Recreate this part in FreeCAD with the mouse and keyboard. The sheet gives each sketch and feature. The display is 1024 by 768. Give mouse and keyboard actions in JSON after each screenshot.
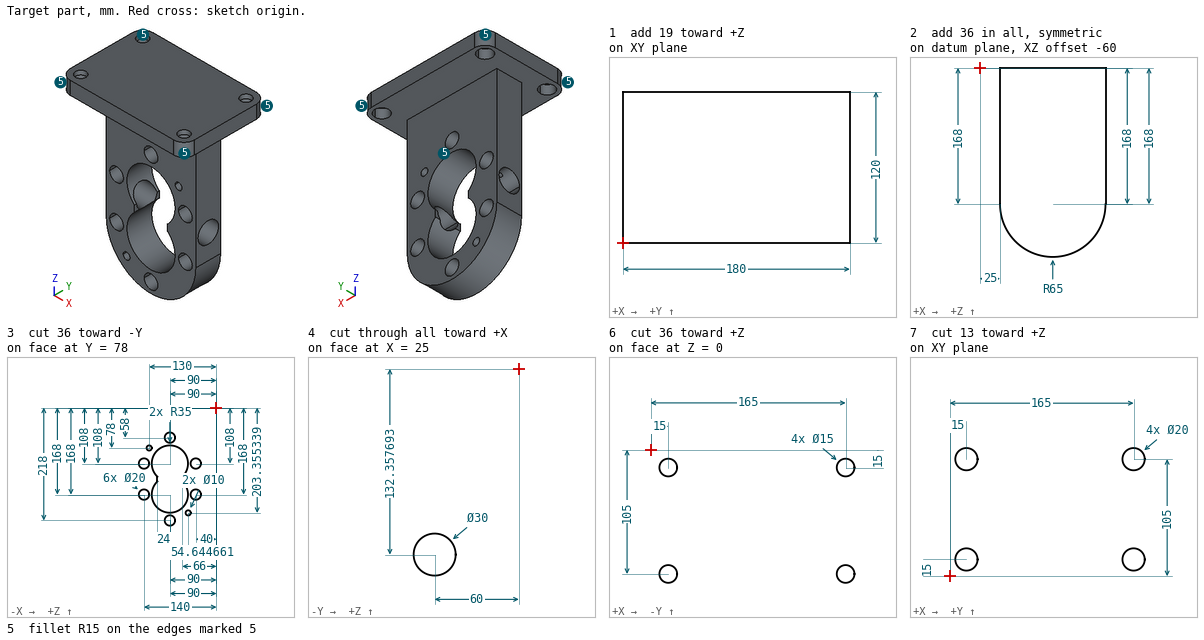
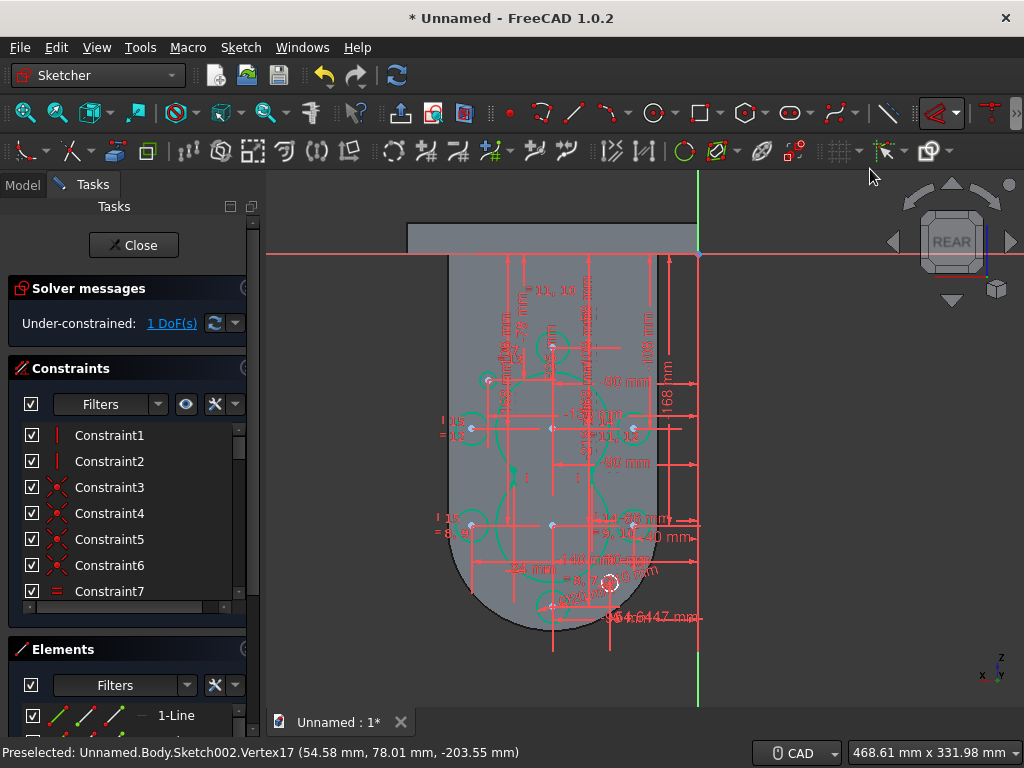
{"action": "left_click", "coordinate": [610, 583]}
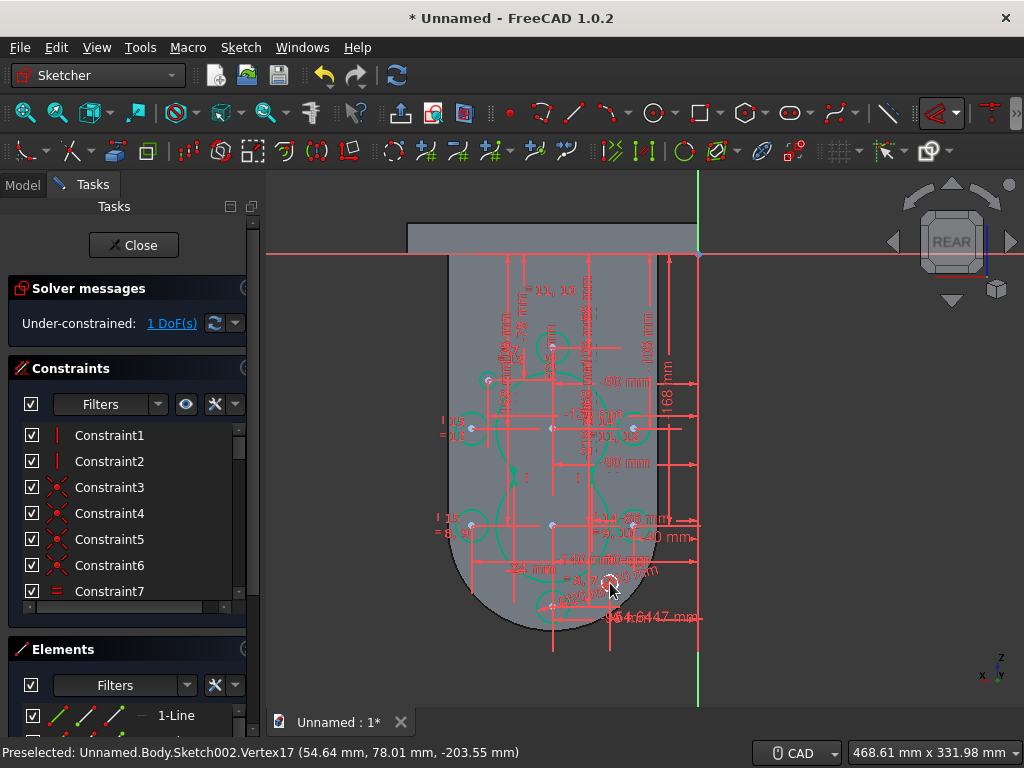
{"action": "left_click", "coordinate": [958, 114]}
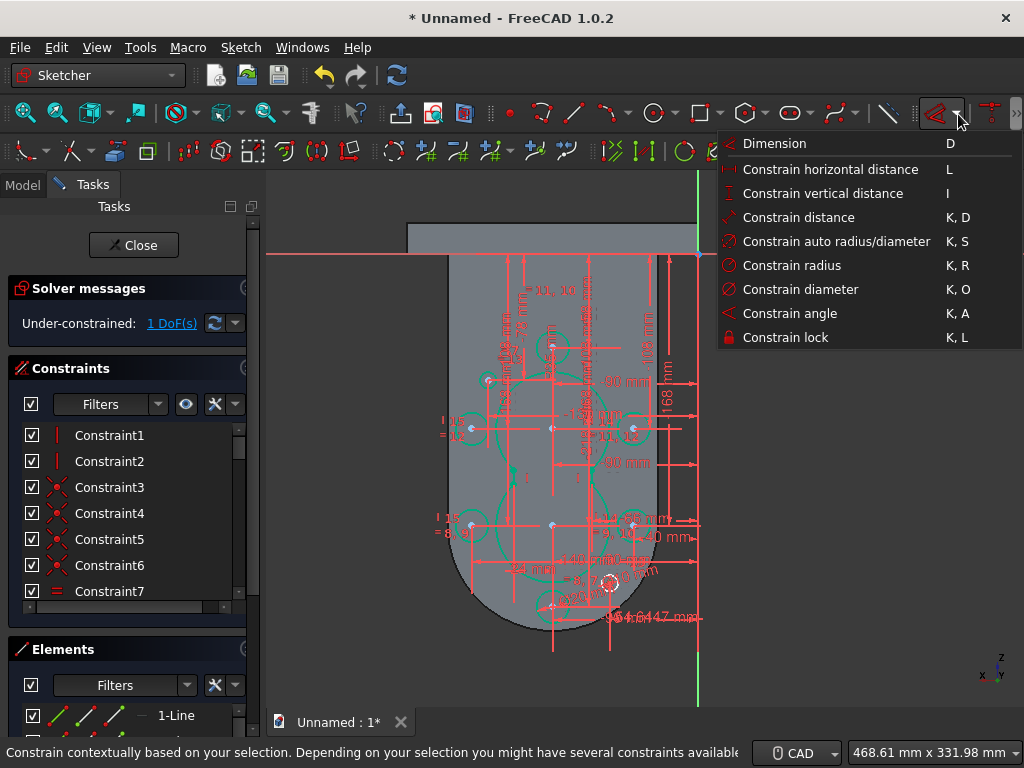
{"action": "left_click", "coordinate": [870, 193]}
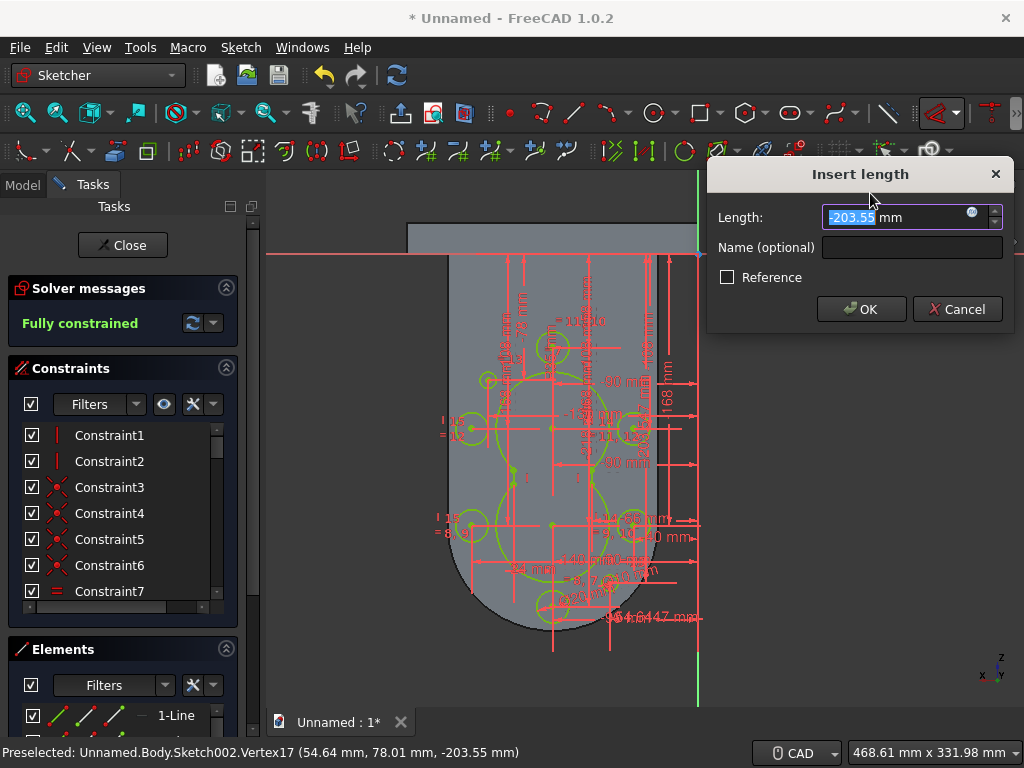
{"action": "type", "text": "-203.355339"}
{"action": "key", "text": "Return"}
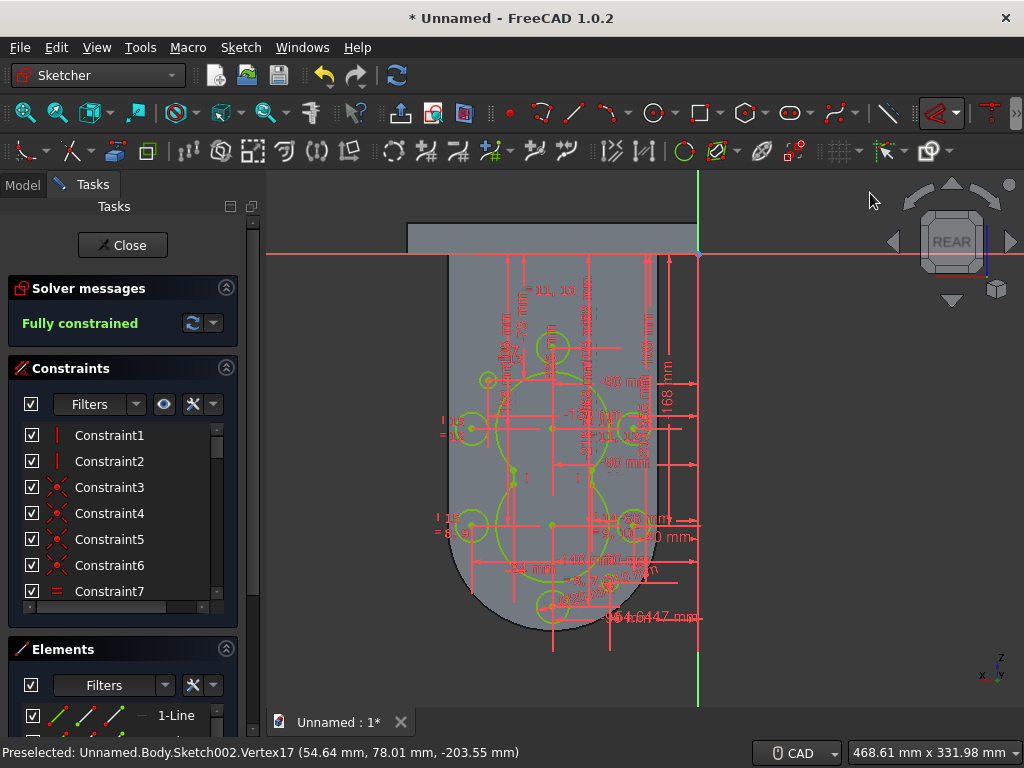
{"action": "left_click", "coordinate": [123, 245]}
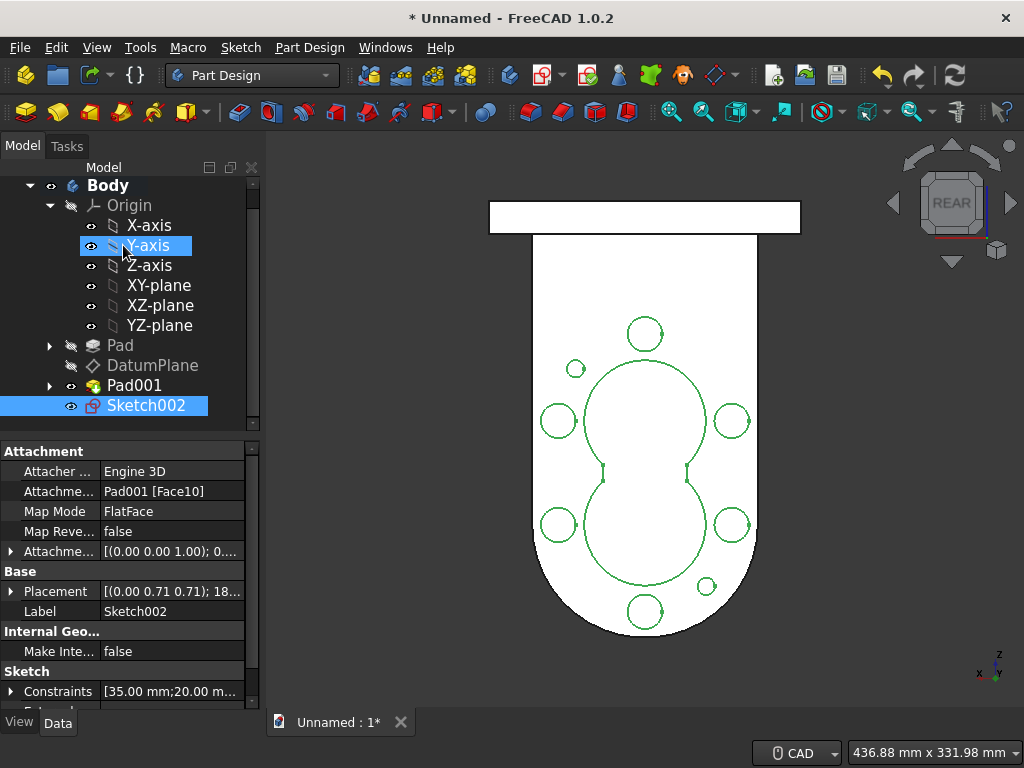
{"action": "left_click", "coordinate": [240, 112]}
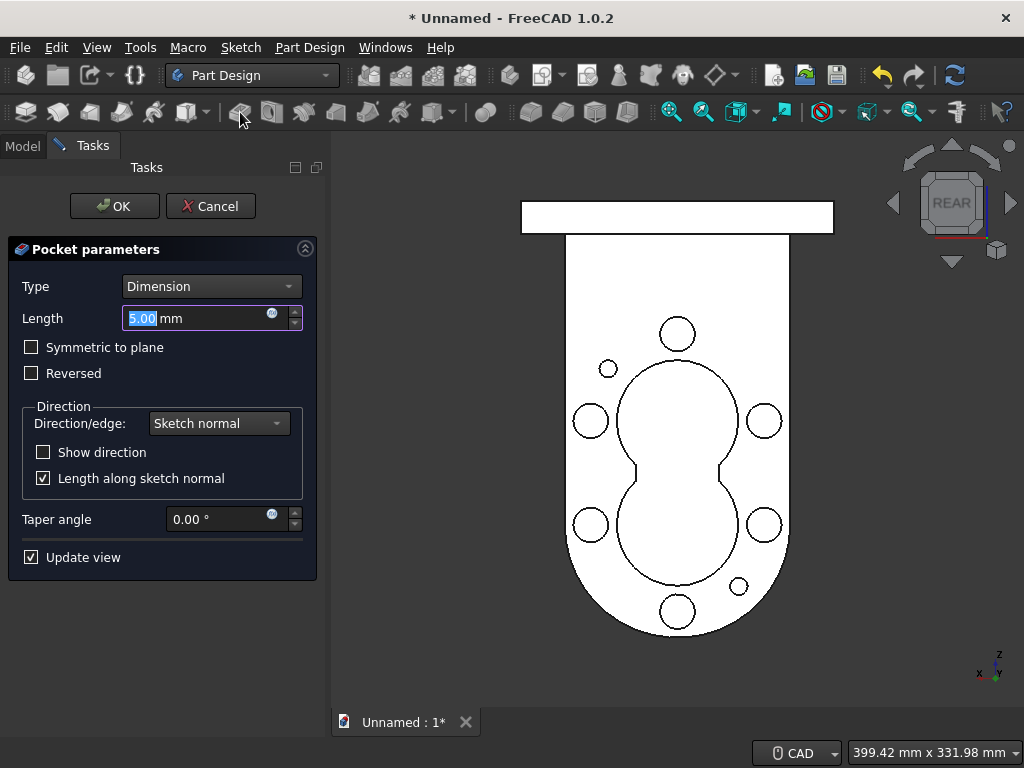
{"action": "type", "text": "36"}
{"action": "key", "text": "Tab"}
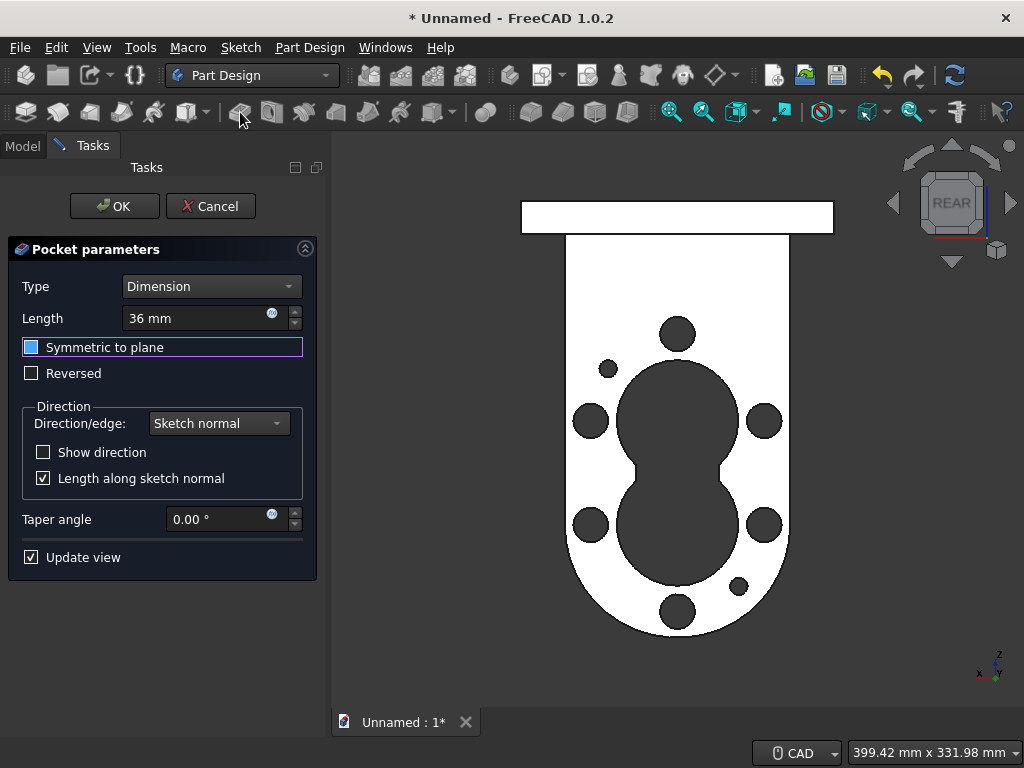
{"action": "left_click", "coordinate": [115, 206]}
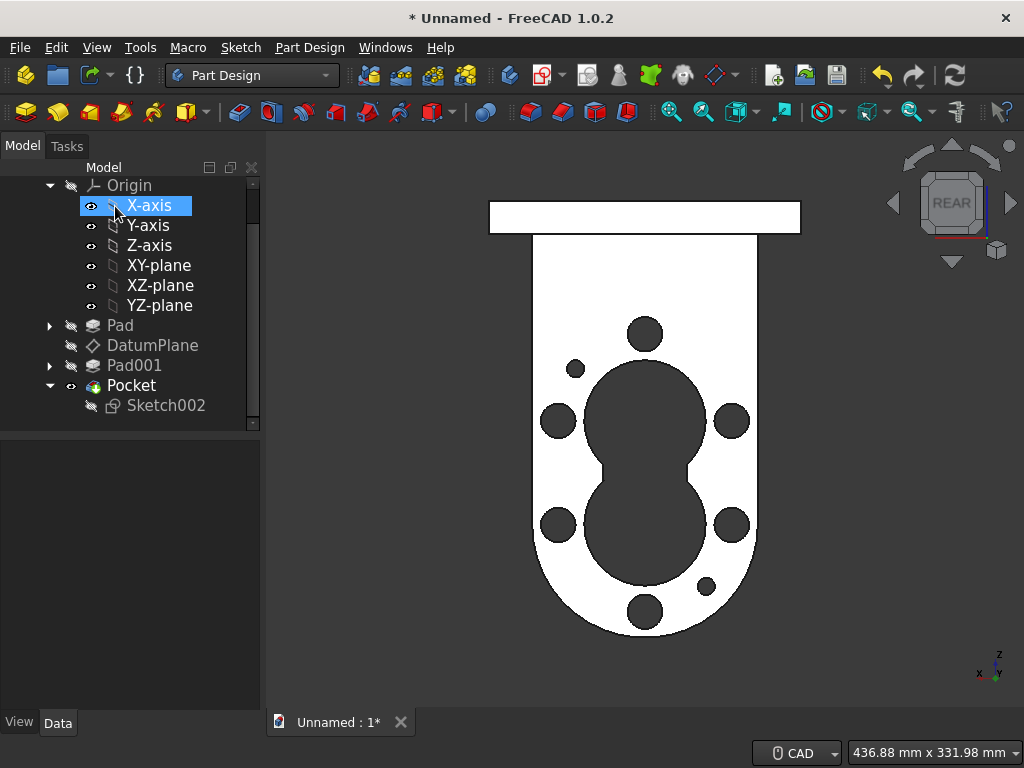
{"action": "key", "text": "6"}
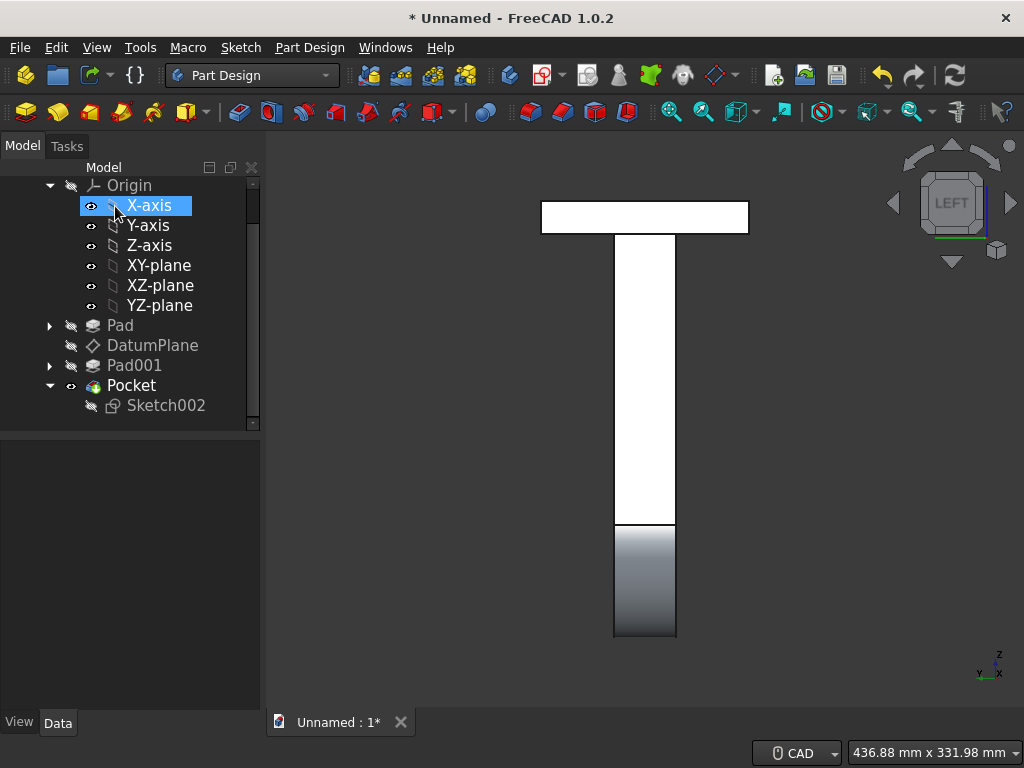
{"action": "left_click", "coordinate": [645, 337]}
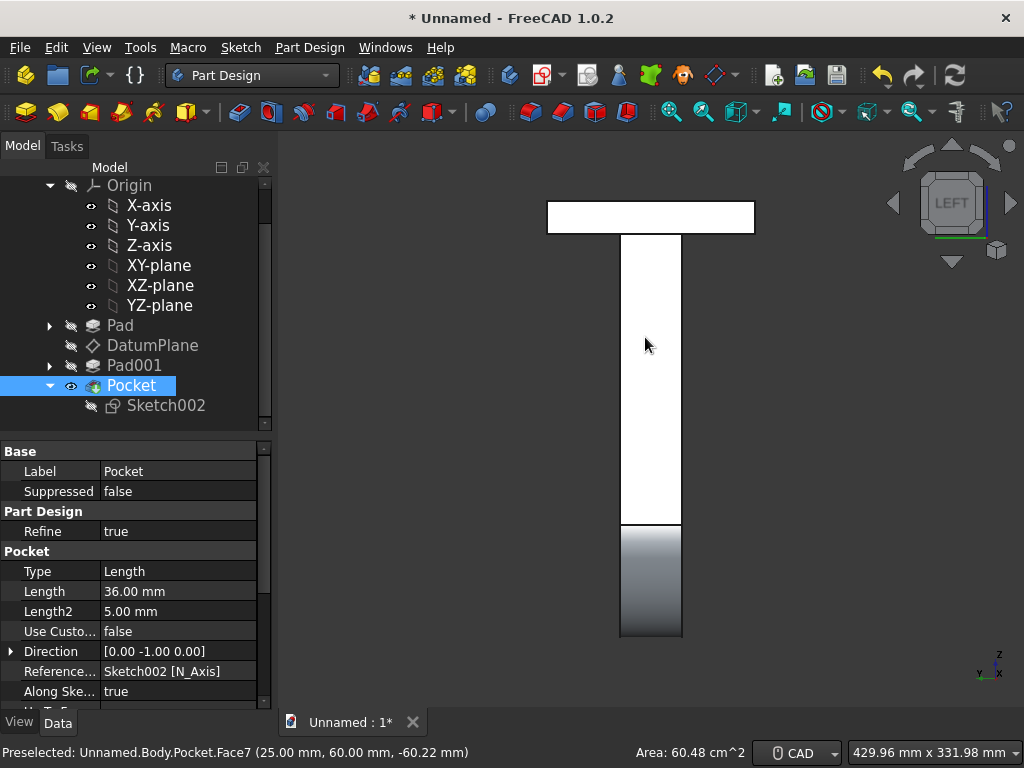
{"action": "left_click", "coordinate": [542, 76]}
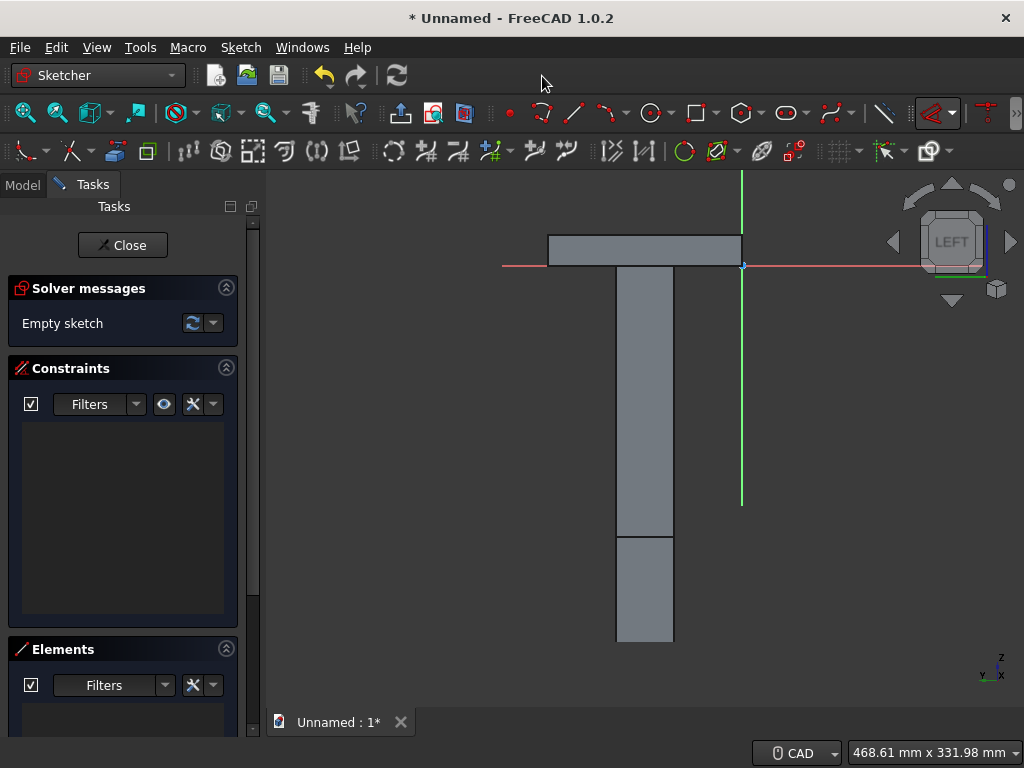
{"action": "left_click", "coordinate": [466, 114]}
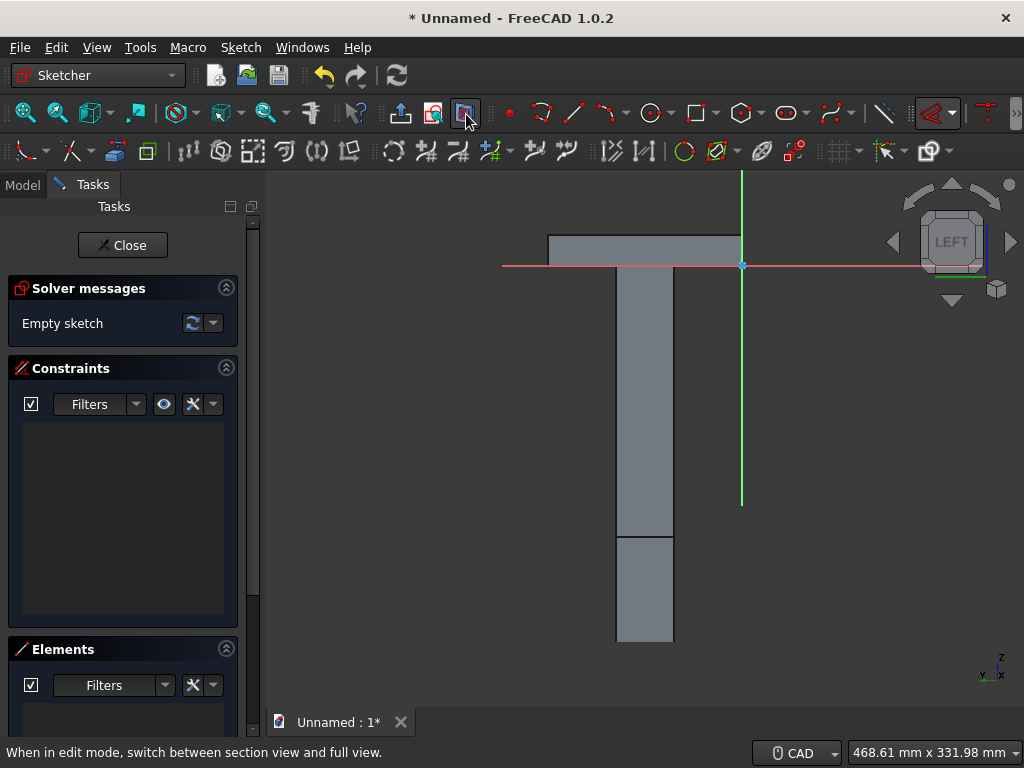
{"action": "scroll", "coordinate": [656, 486], "scroll_direction": "up", "scroll_amount": 10}